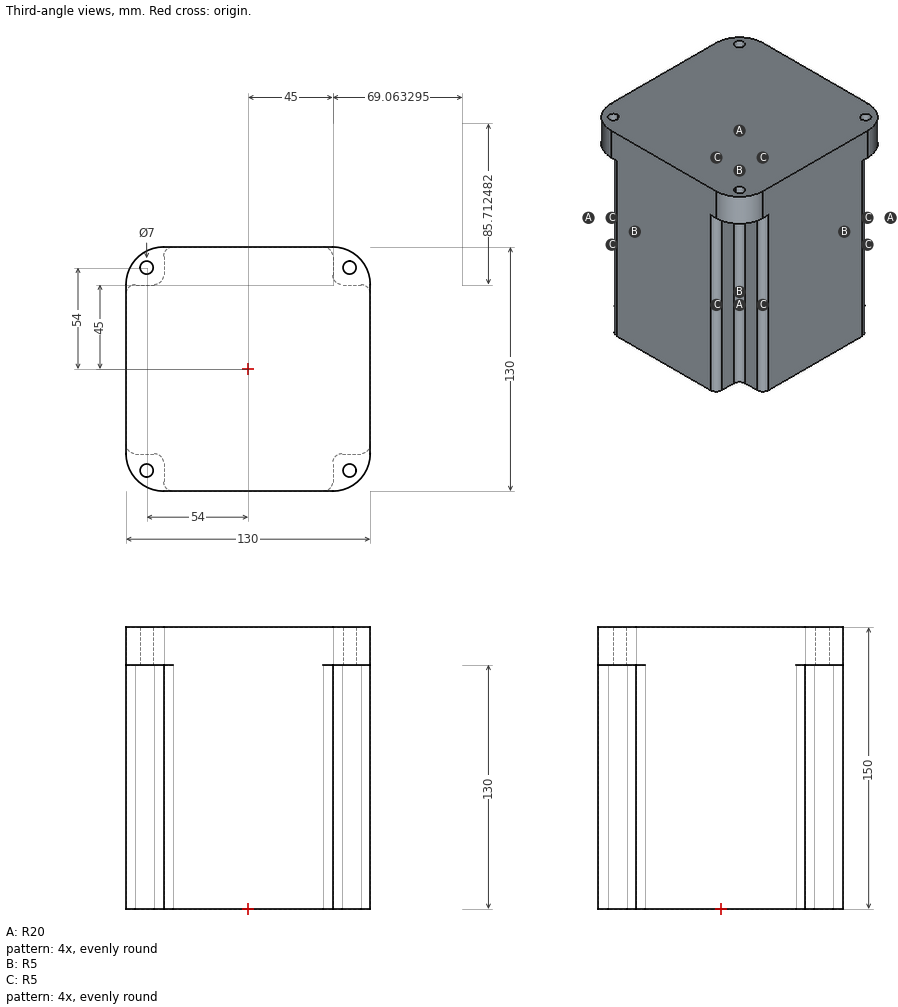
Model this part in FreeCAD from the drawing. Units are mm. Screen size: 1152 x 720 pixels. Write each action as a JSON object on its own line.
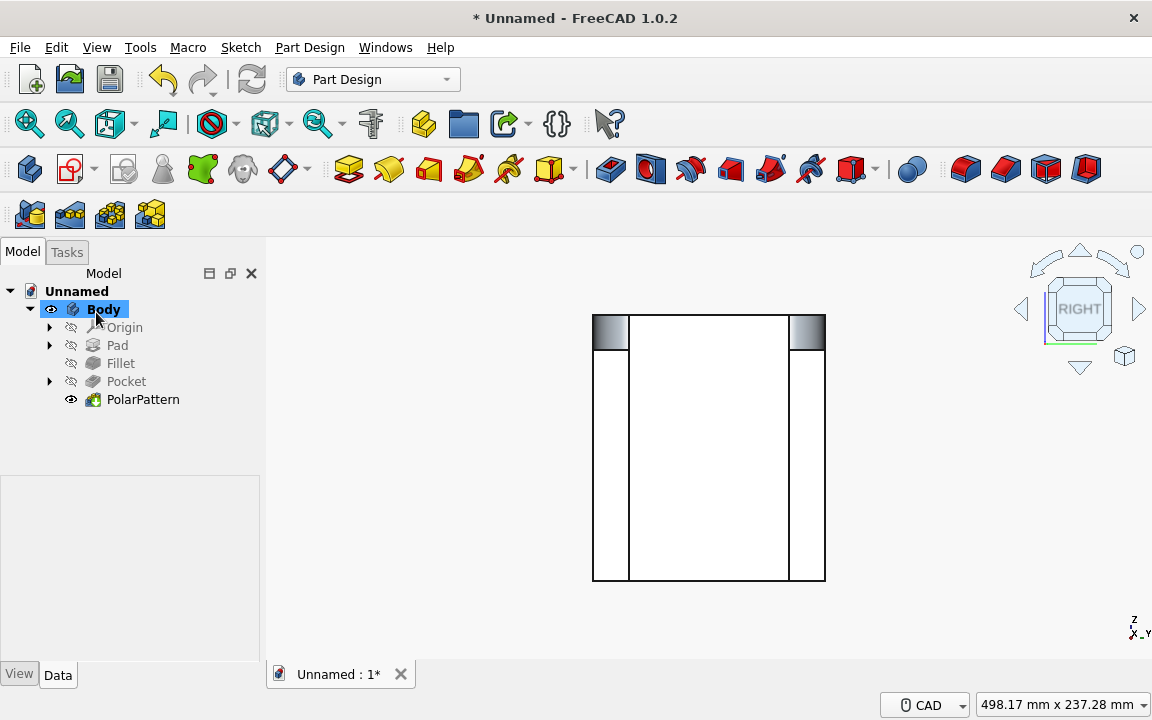
{"action": "key", "text": "5"}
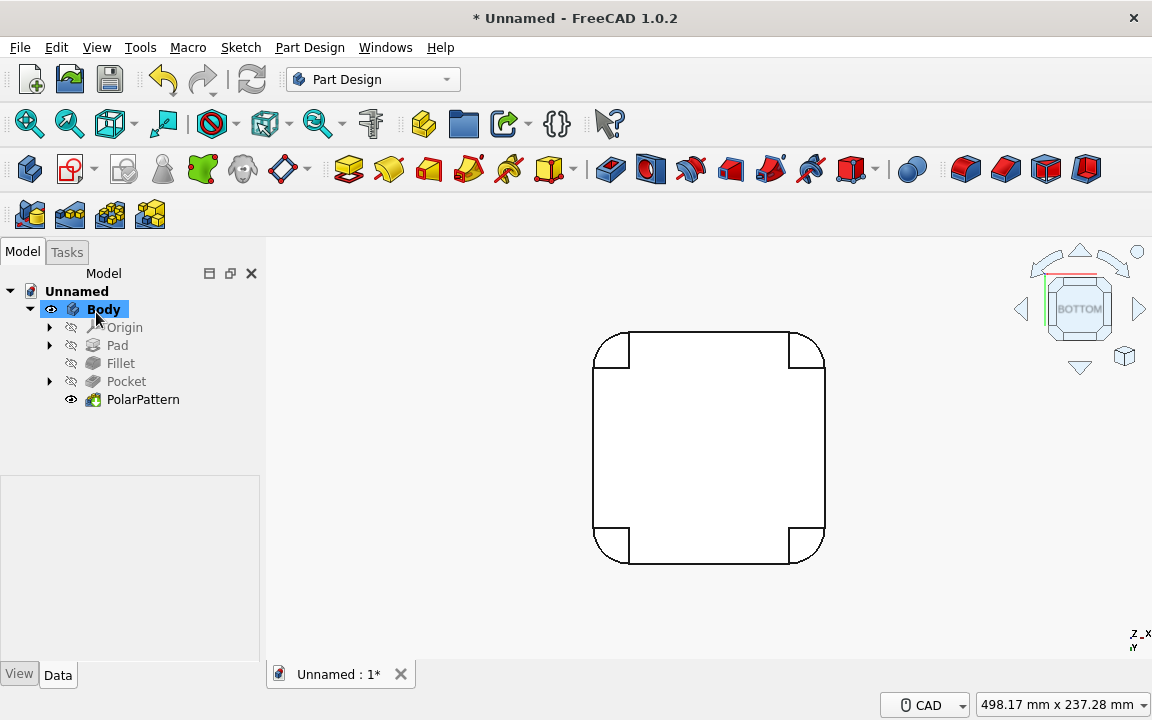
{"action": "key", "text": "4"}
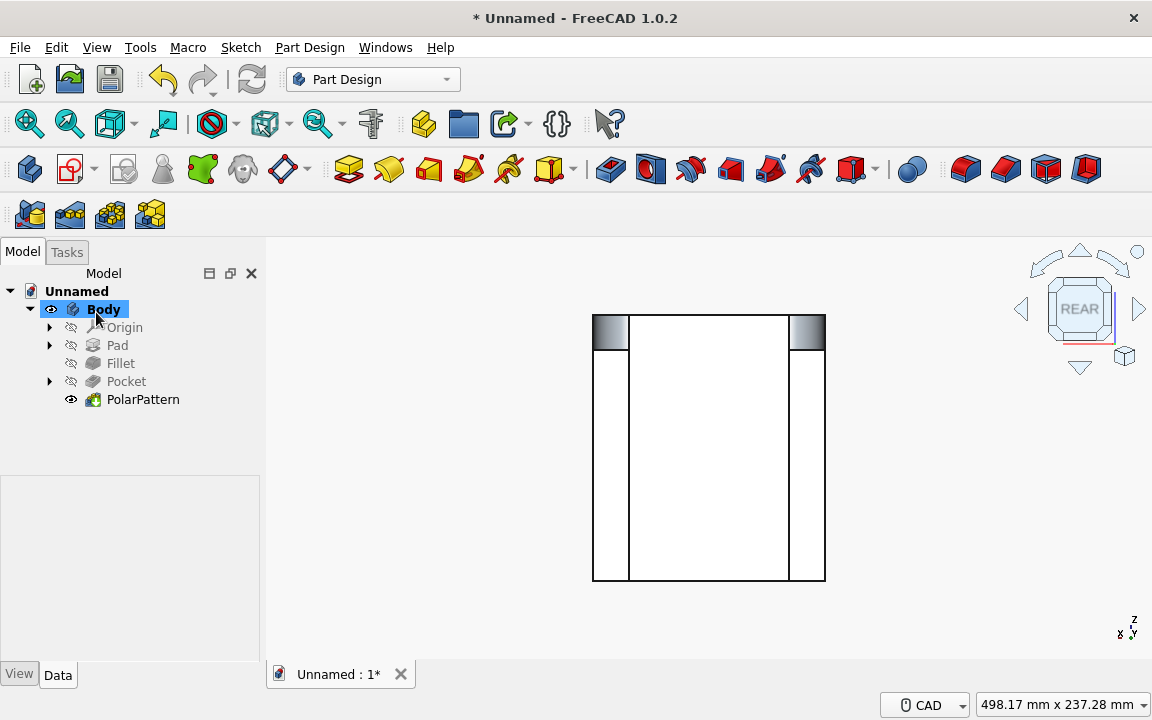
{"action": "key", "text": "6"}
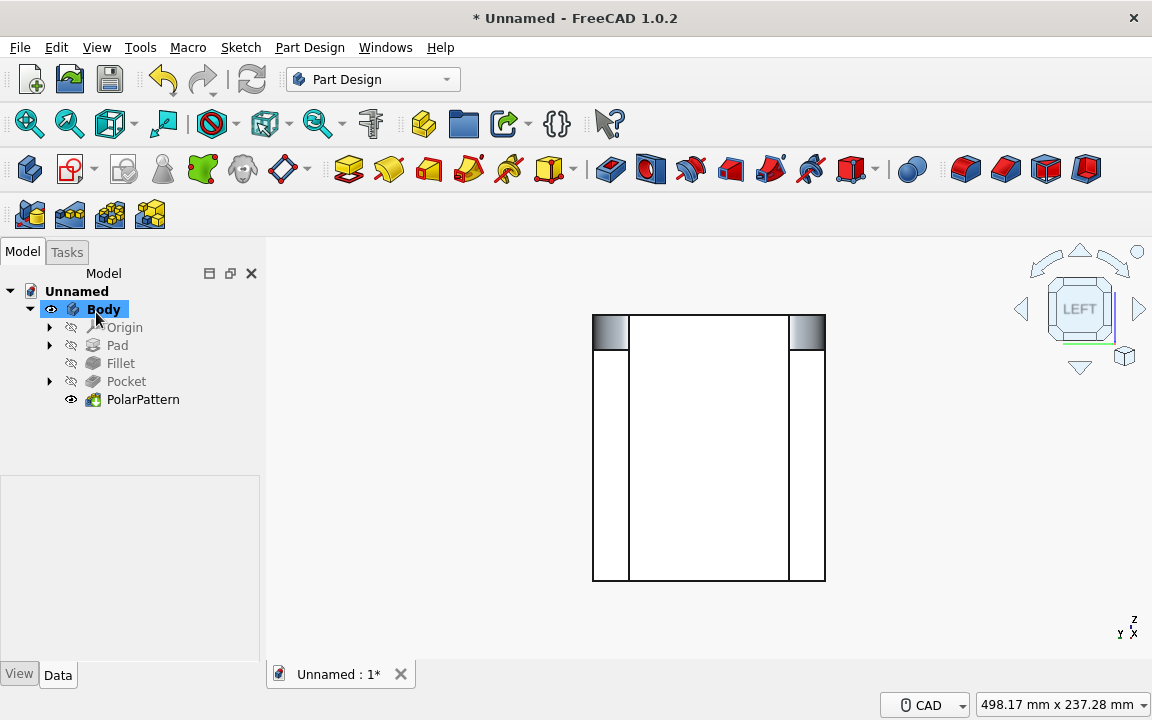
{"action": "key", "text": "v 3"}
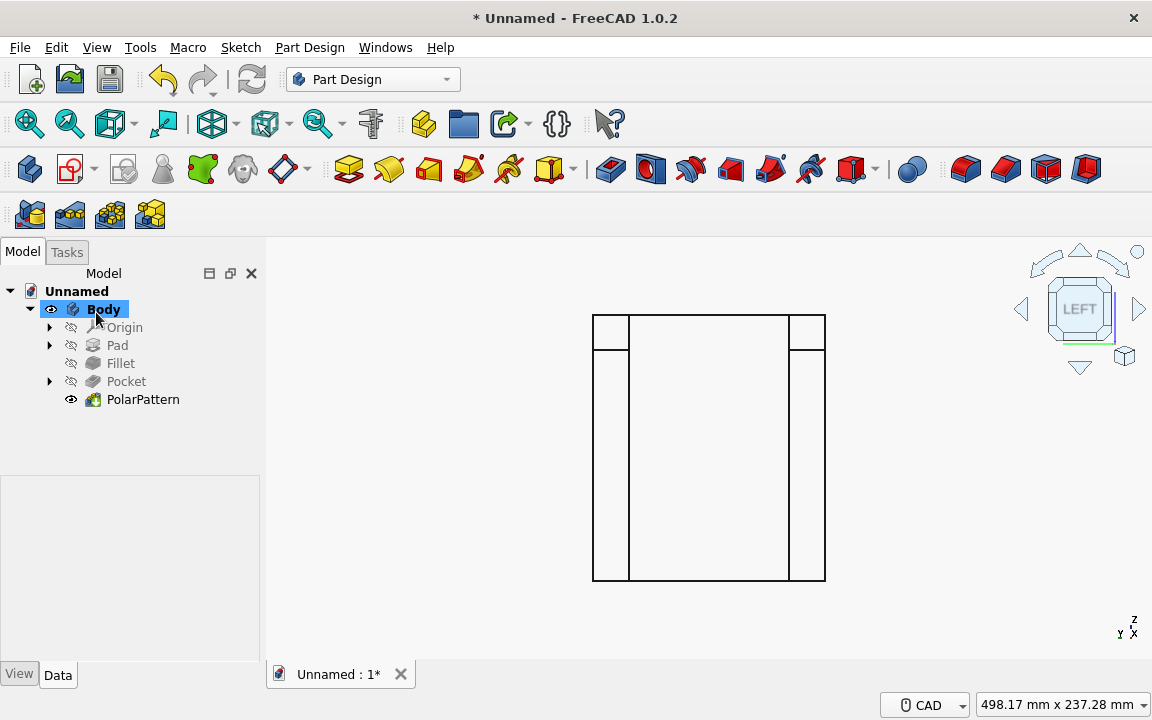
{"action": "key", "text": "0"}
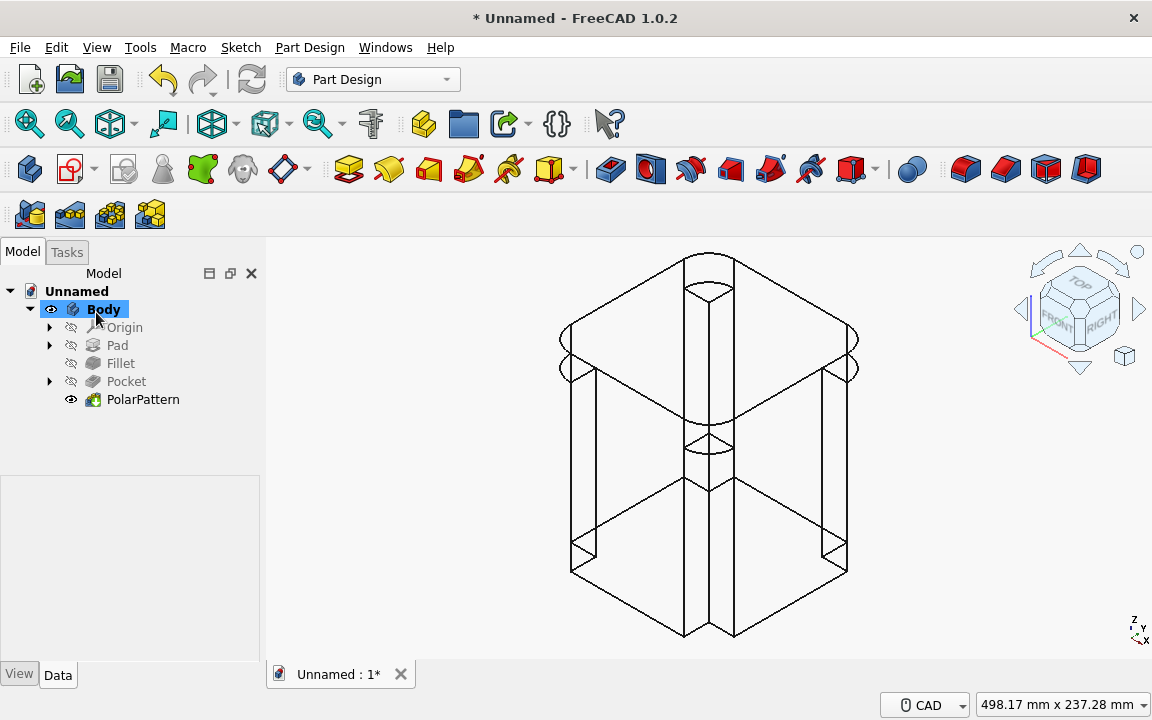
{"action": "left_click", "coordinate": [822, 462]}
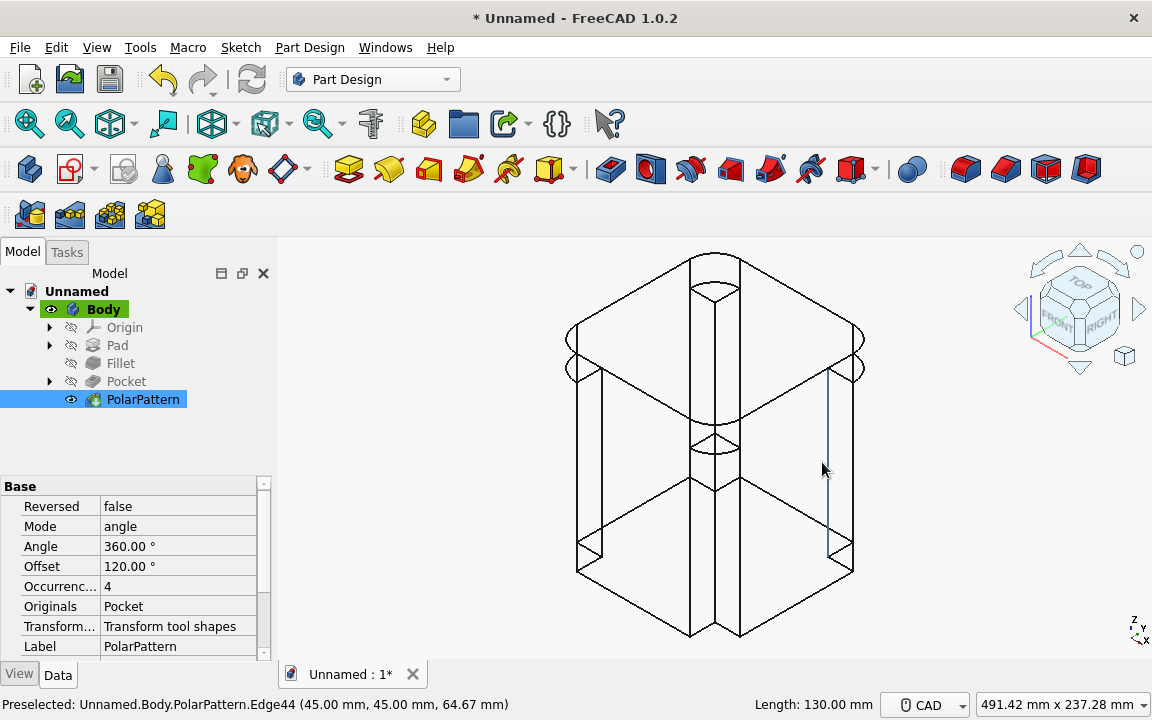
{"action": "left_click", "coordinate": [715, 396], "text": "ctrl"}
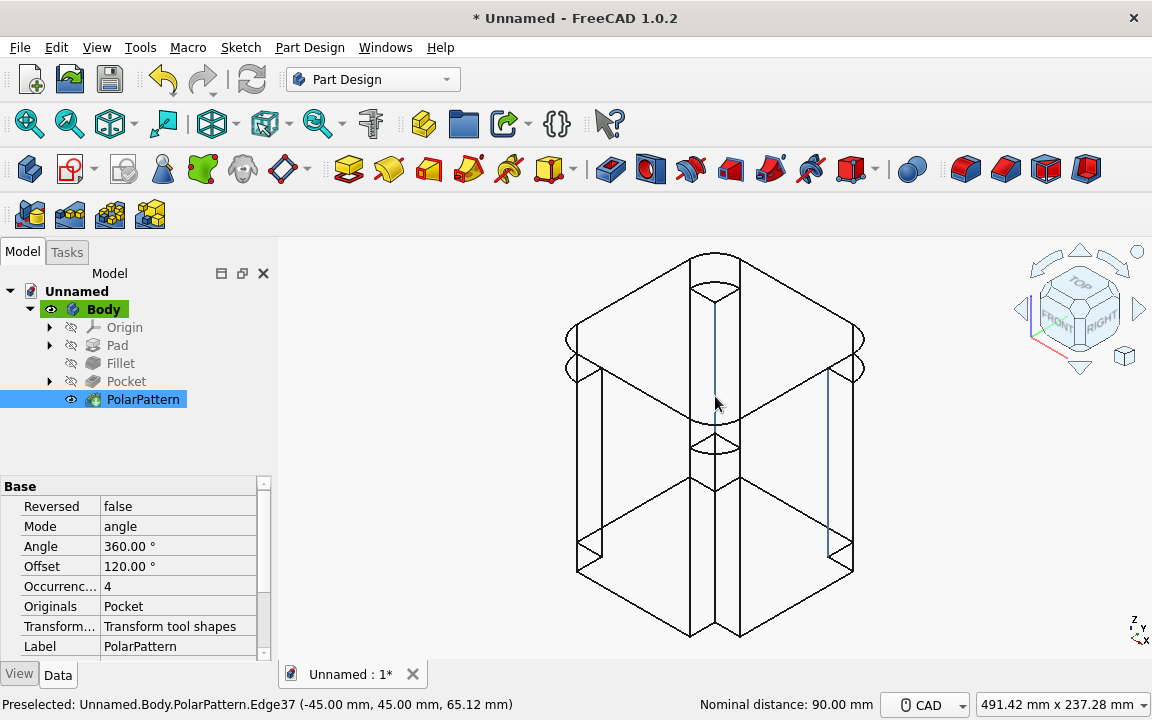
{"action": "left_click", "coordinate": [602, 462], "text": "ctrl"}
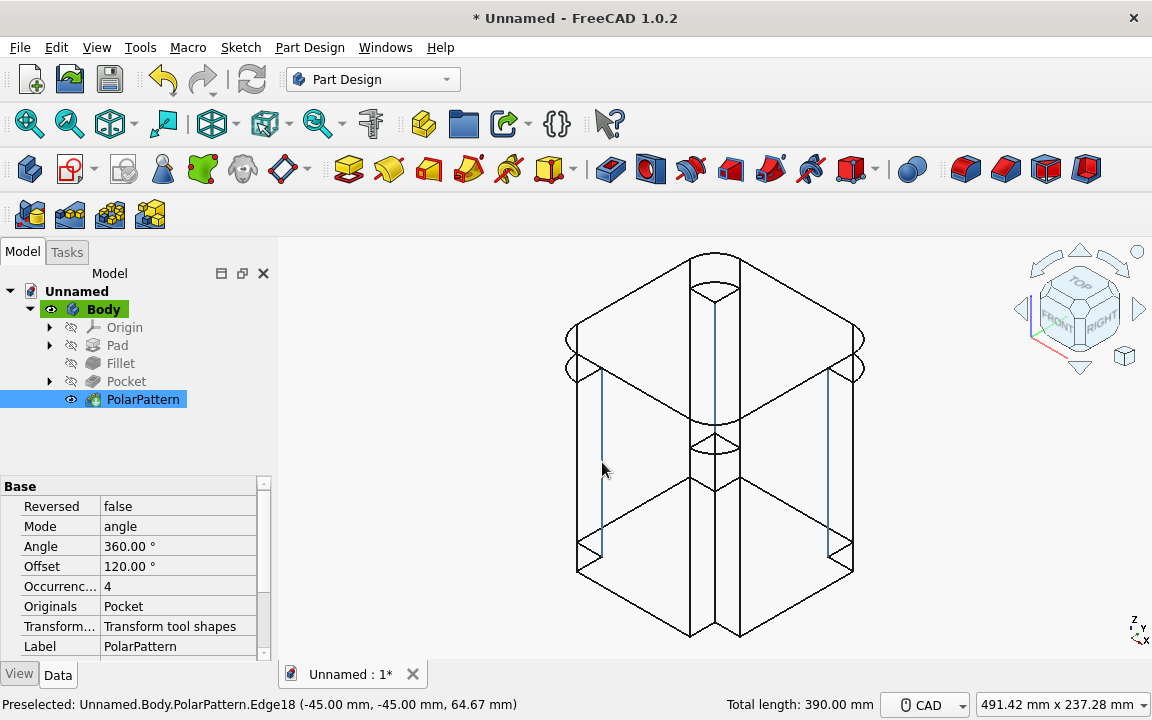
{"action": "left_click", "coordinate": [715, 527], "text": "ctrl"}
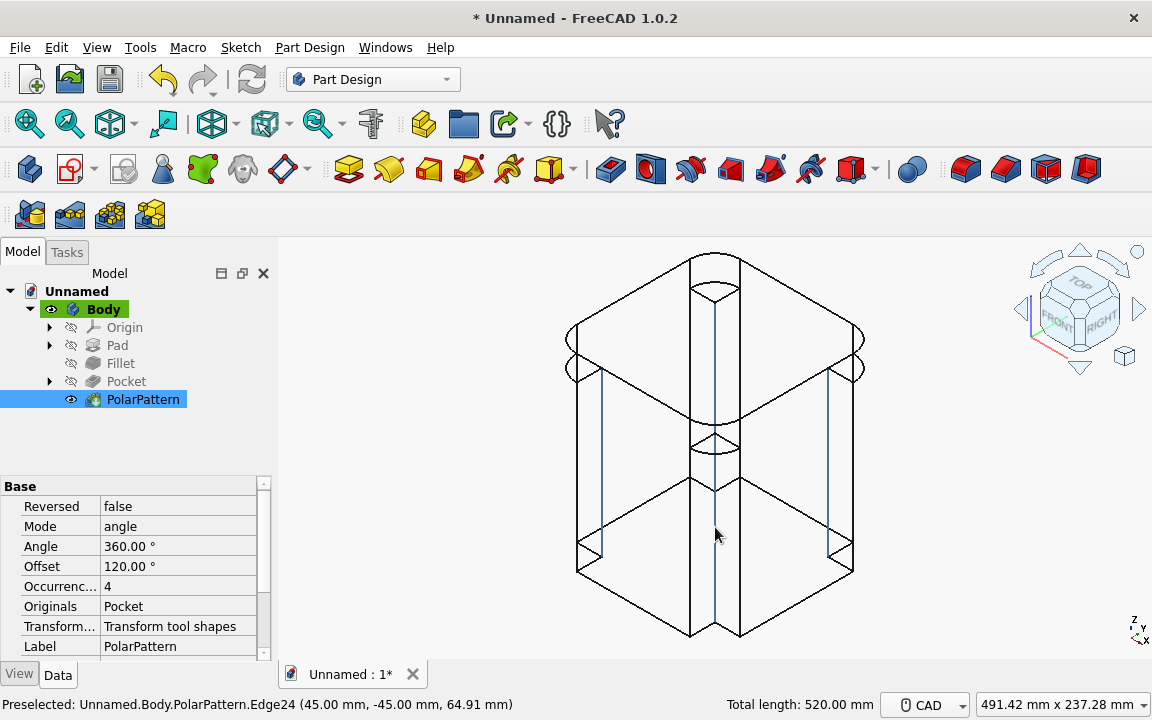
{"action": "key", "text": "v 1"}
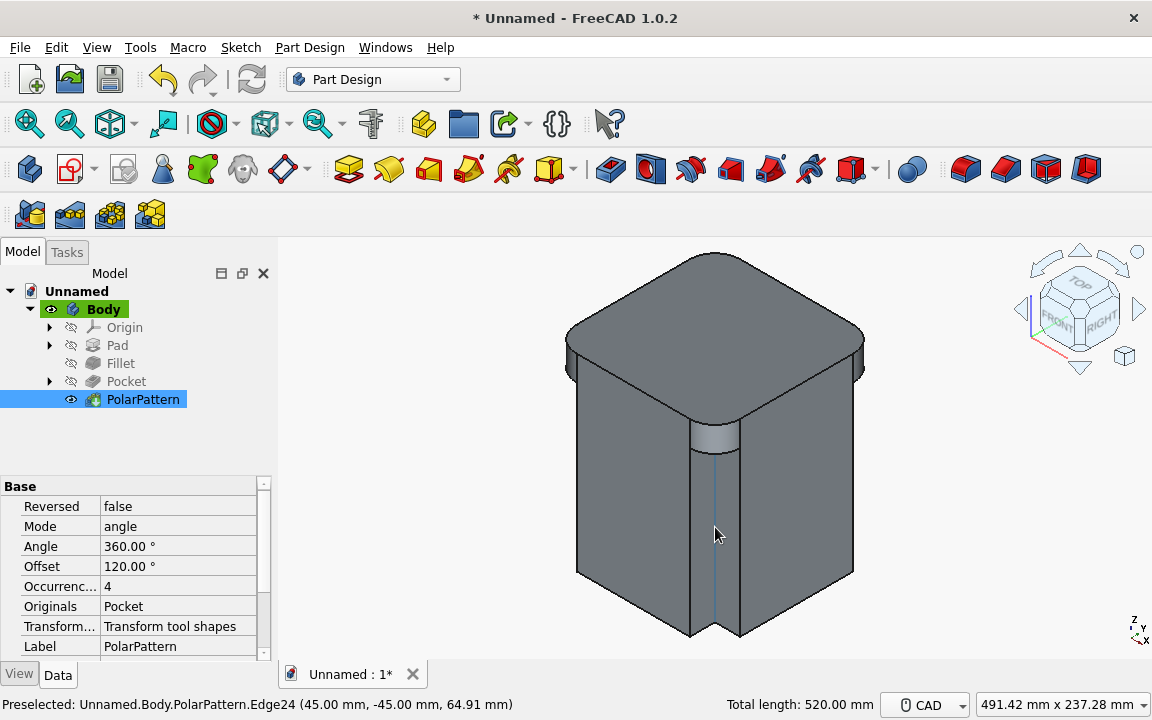
{"action": "left_click", "coordinate": [966, 170]}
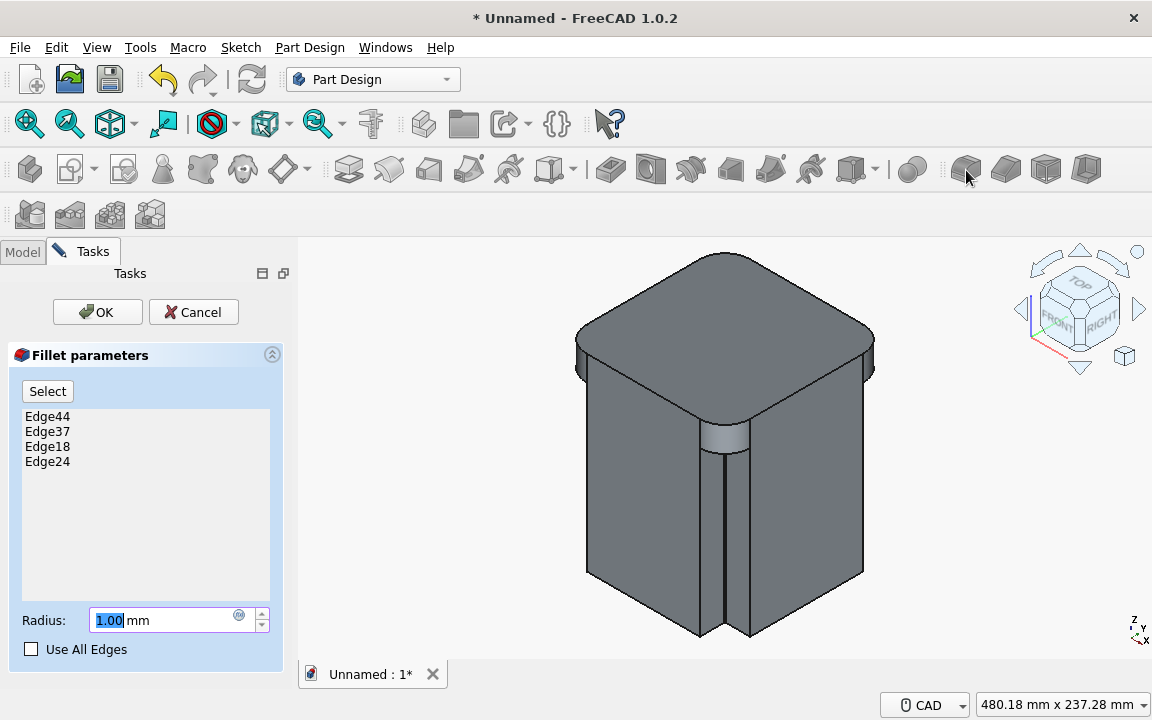
{"action": "type", "text": "5"}
{"action": "key", "text": "Tab"}